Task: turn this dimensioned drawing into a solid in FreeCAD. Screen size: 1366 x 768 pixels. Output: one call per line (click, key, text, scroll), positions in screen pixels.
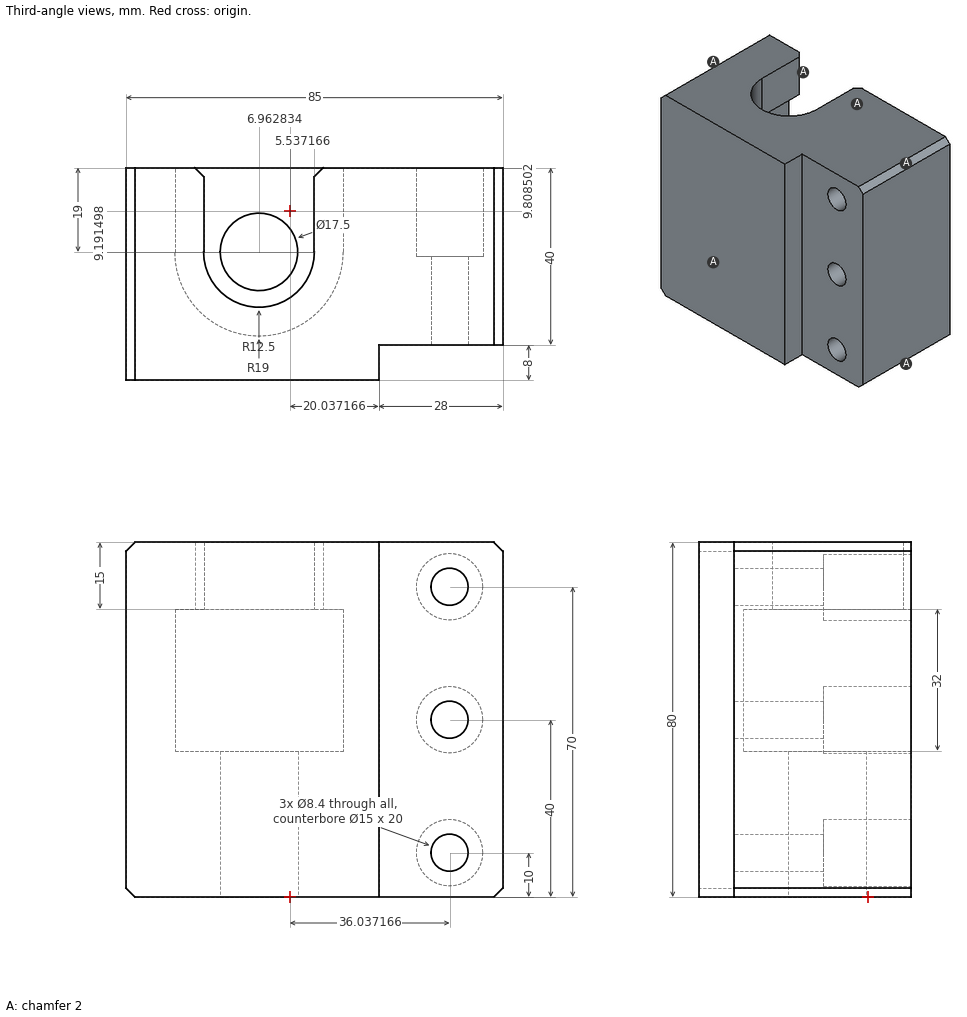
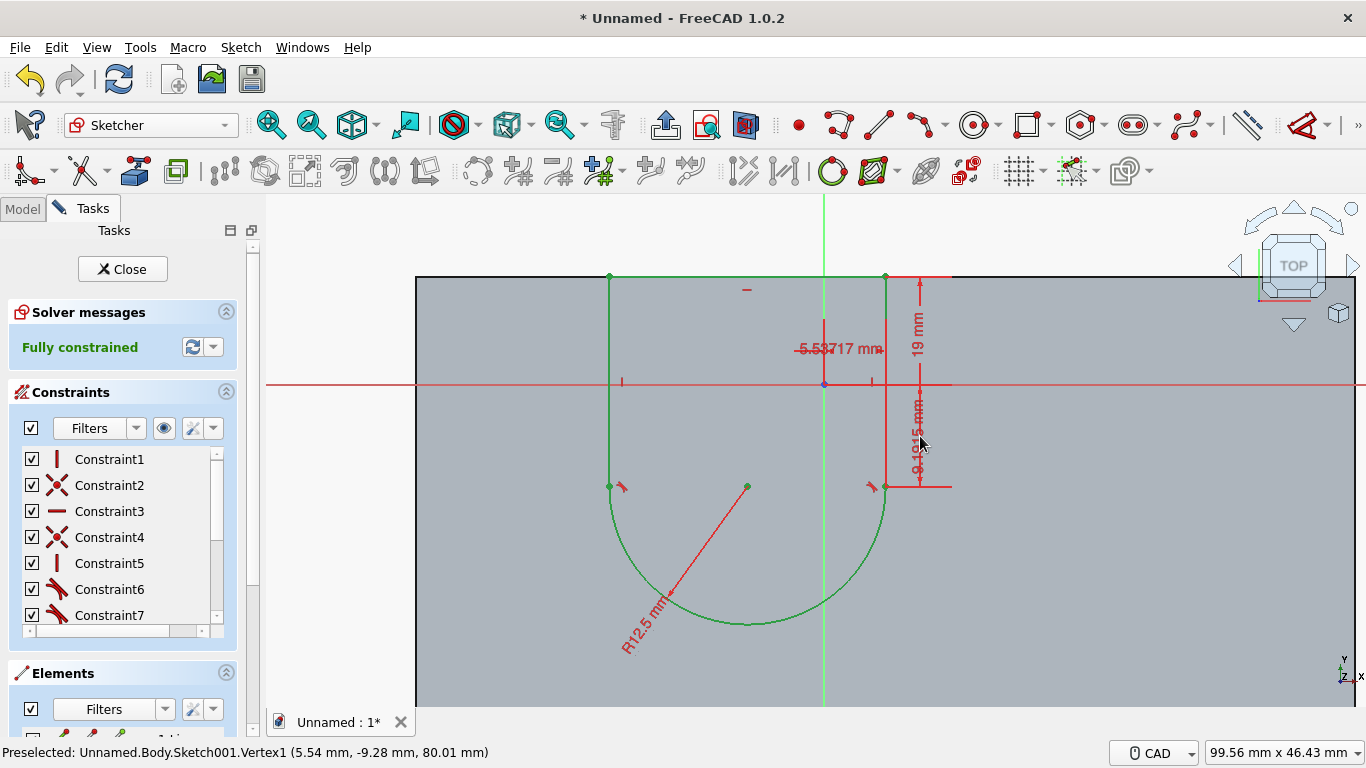
click(123, 269)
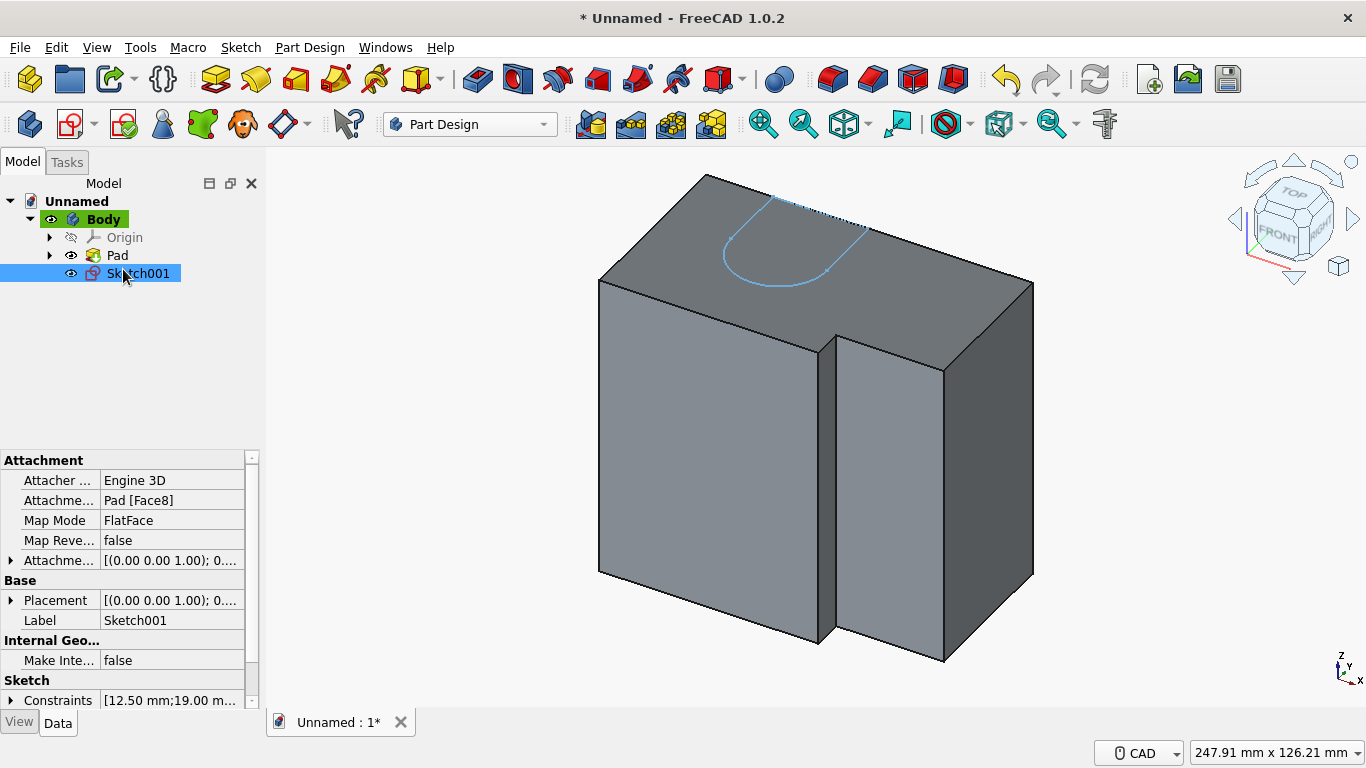
click(478, 80)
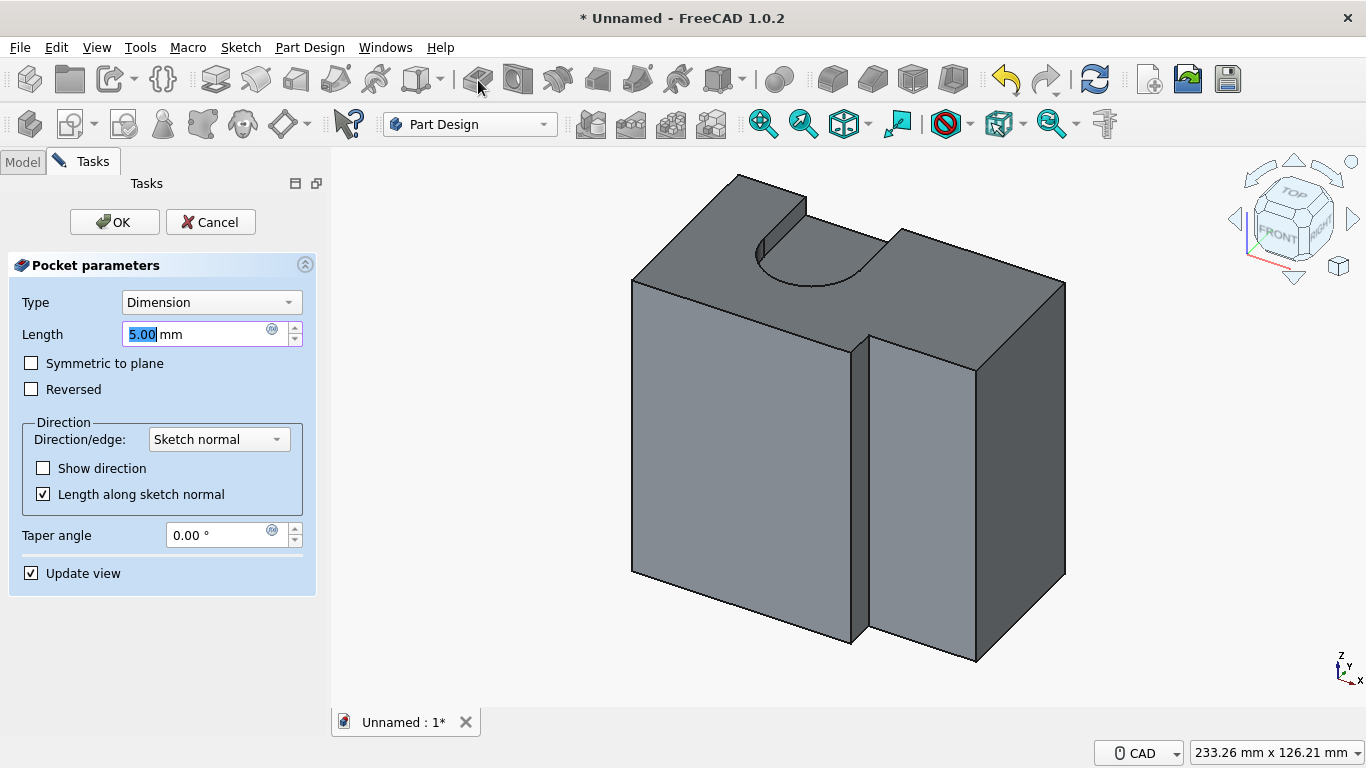
text(15)
key(Tab)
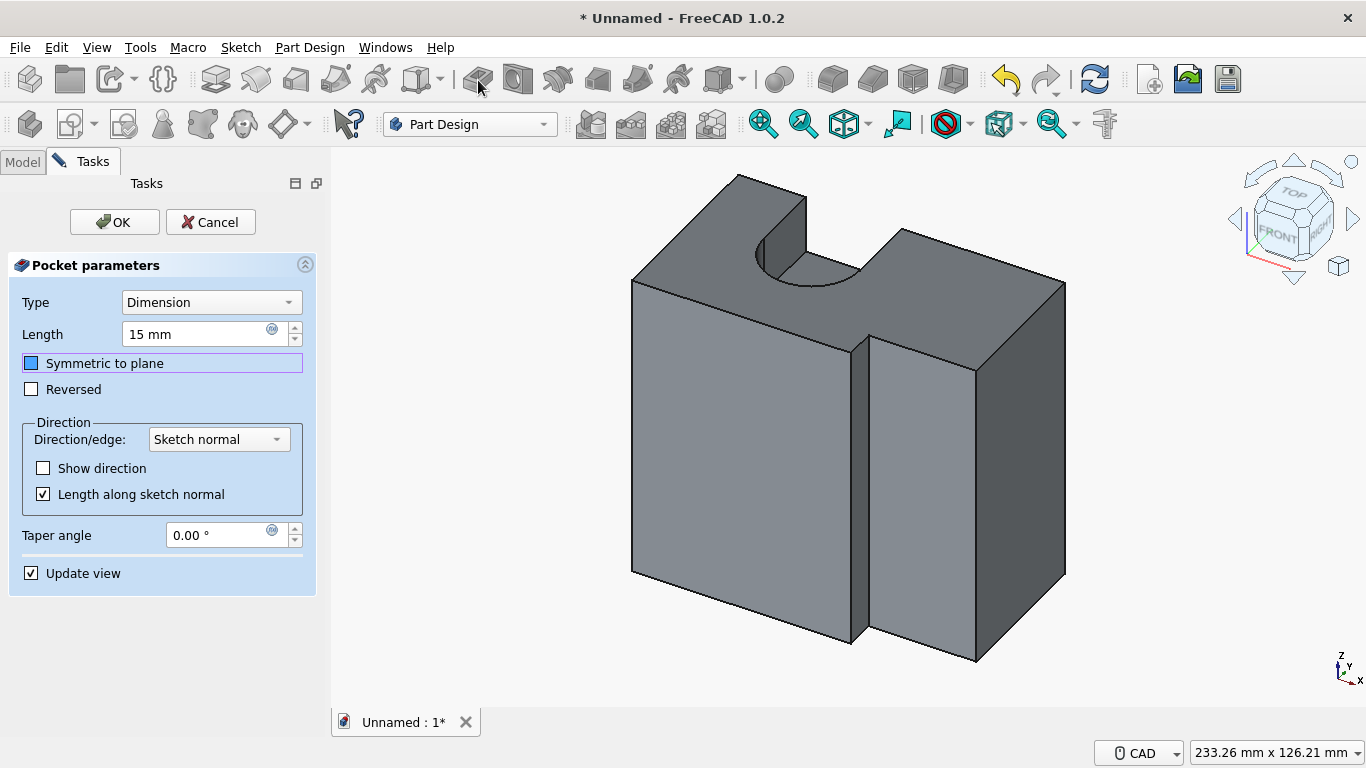
click(115, 222)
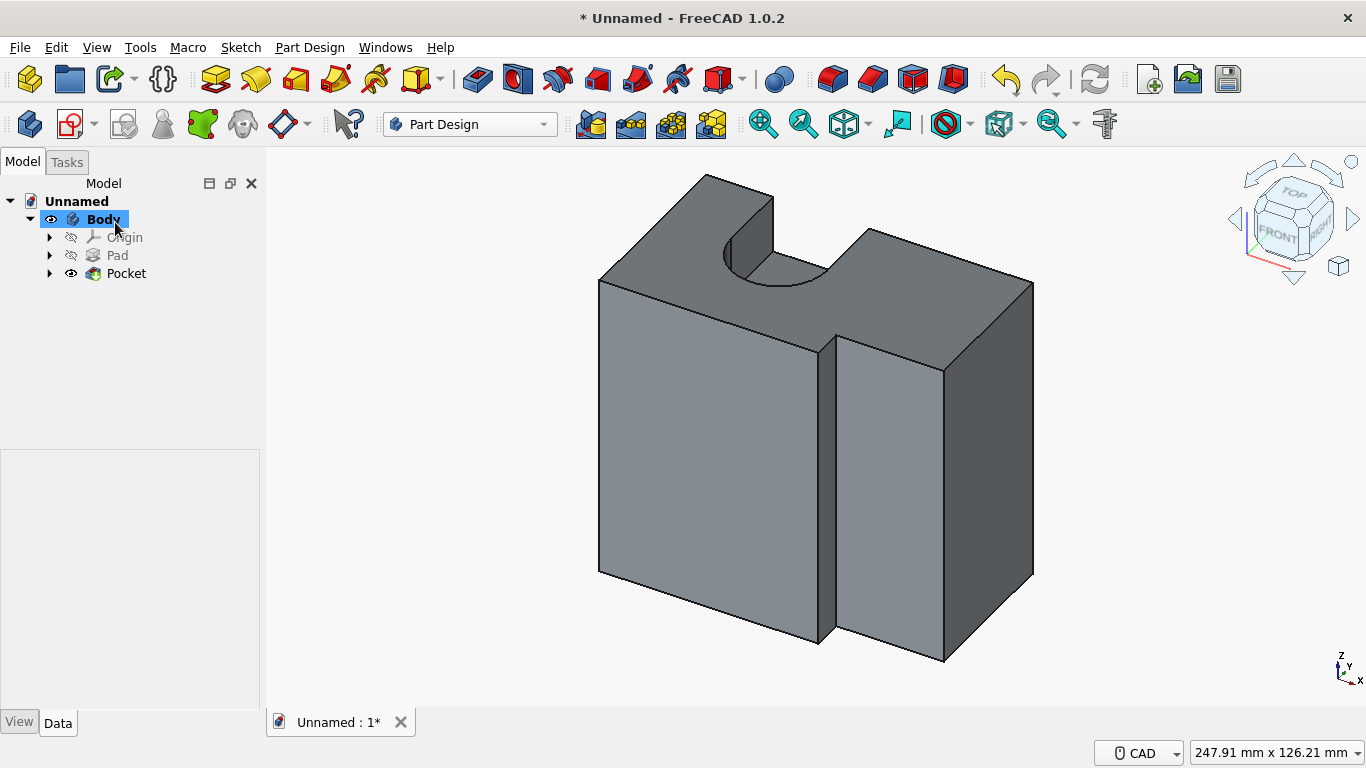
key(0)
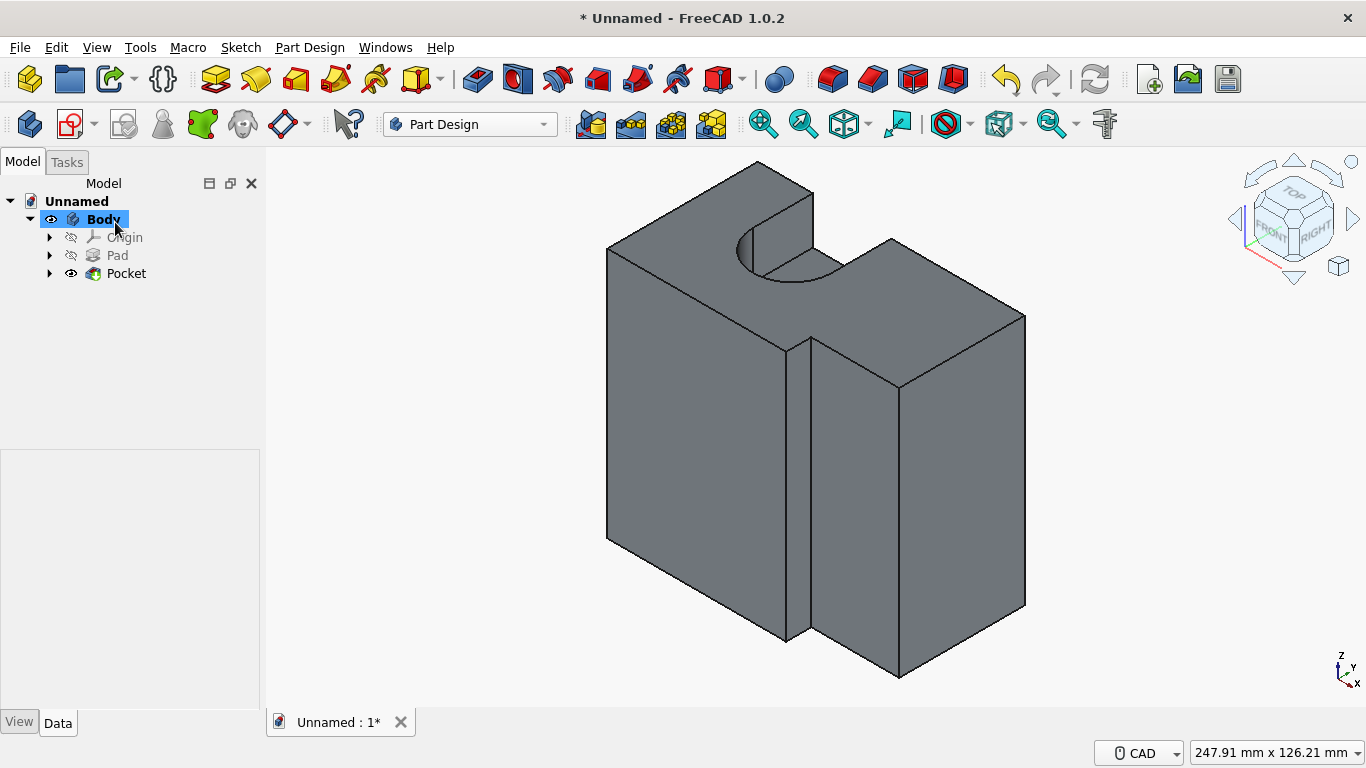
key(2)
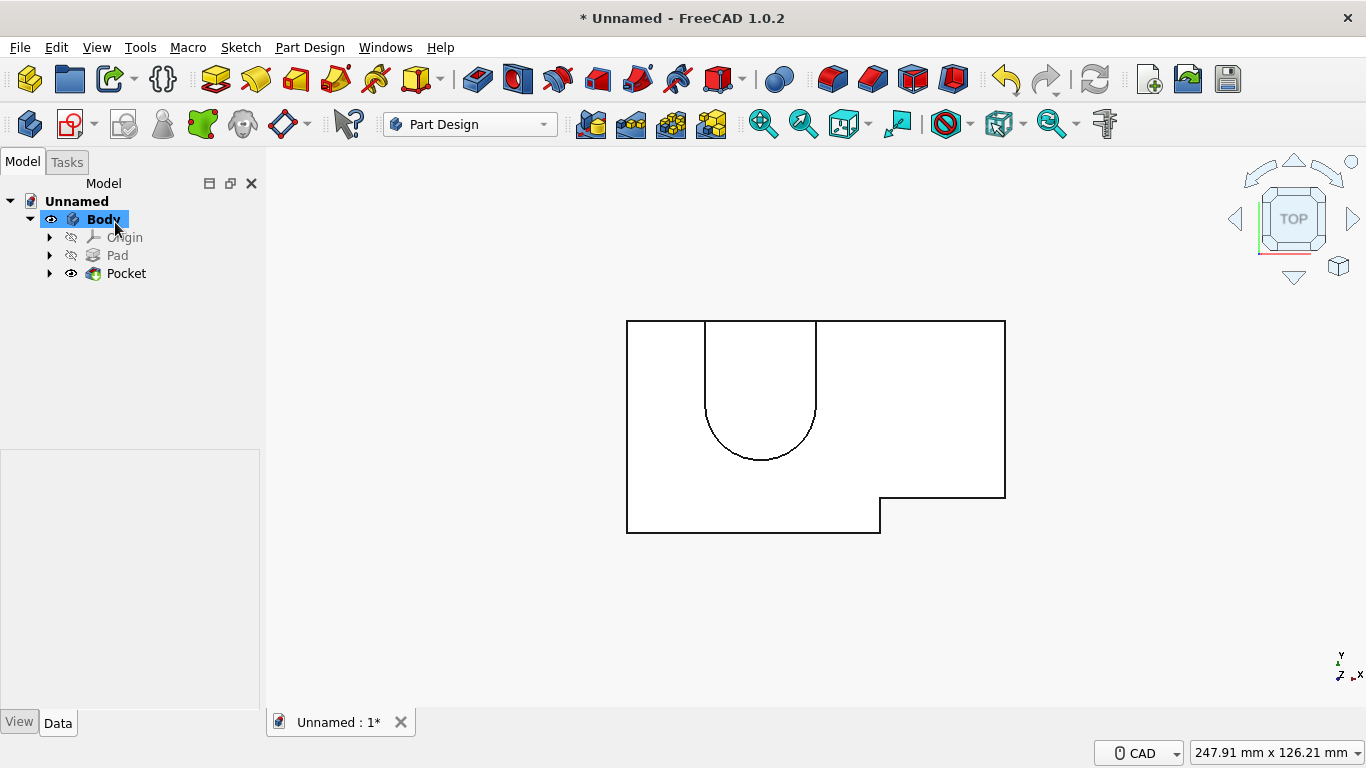
click(764, 124)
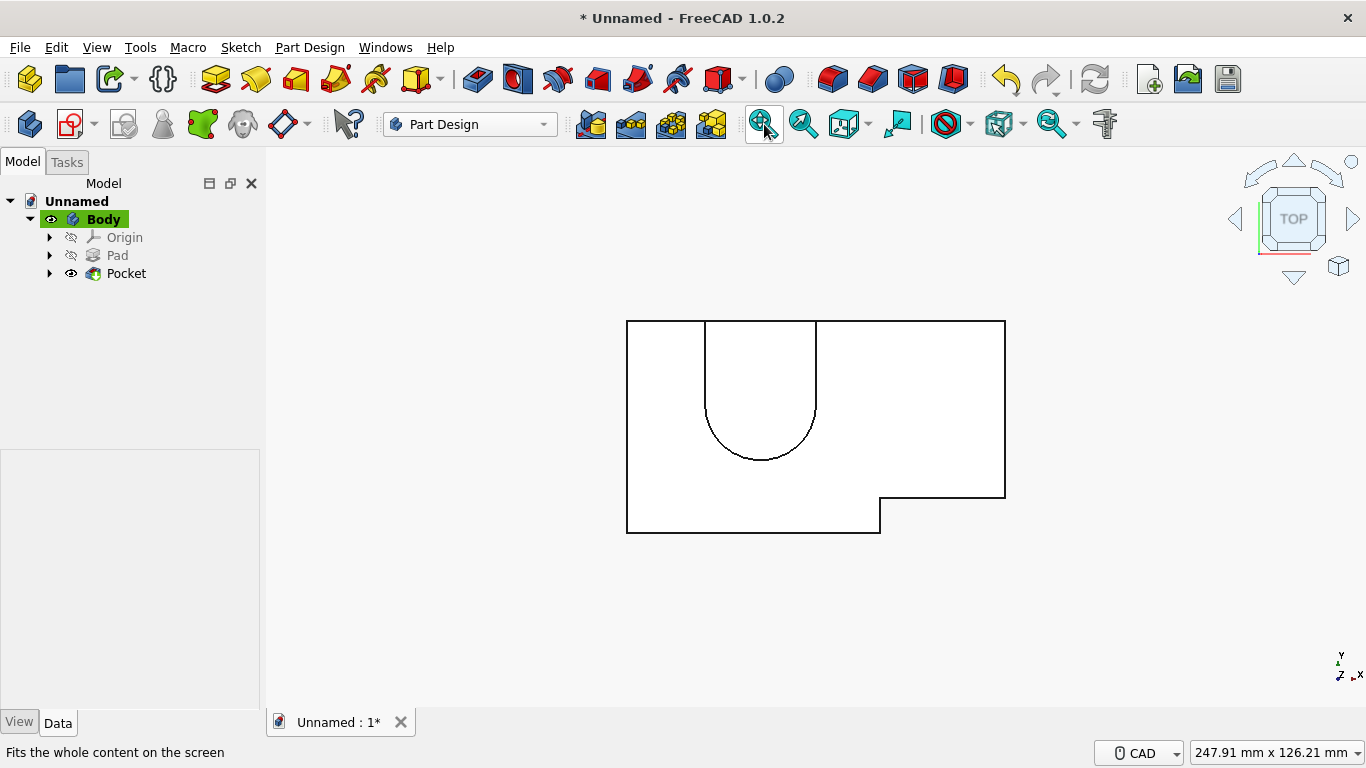
click(761, 389)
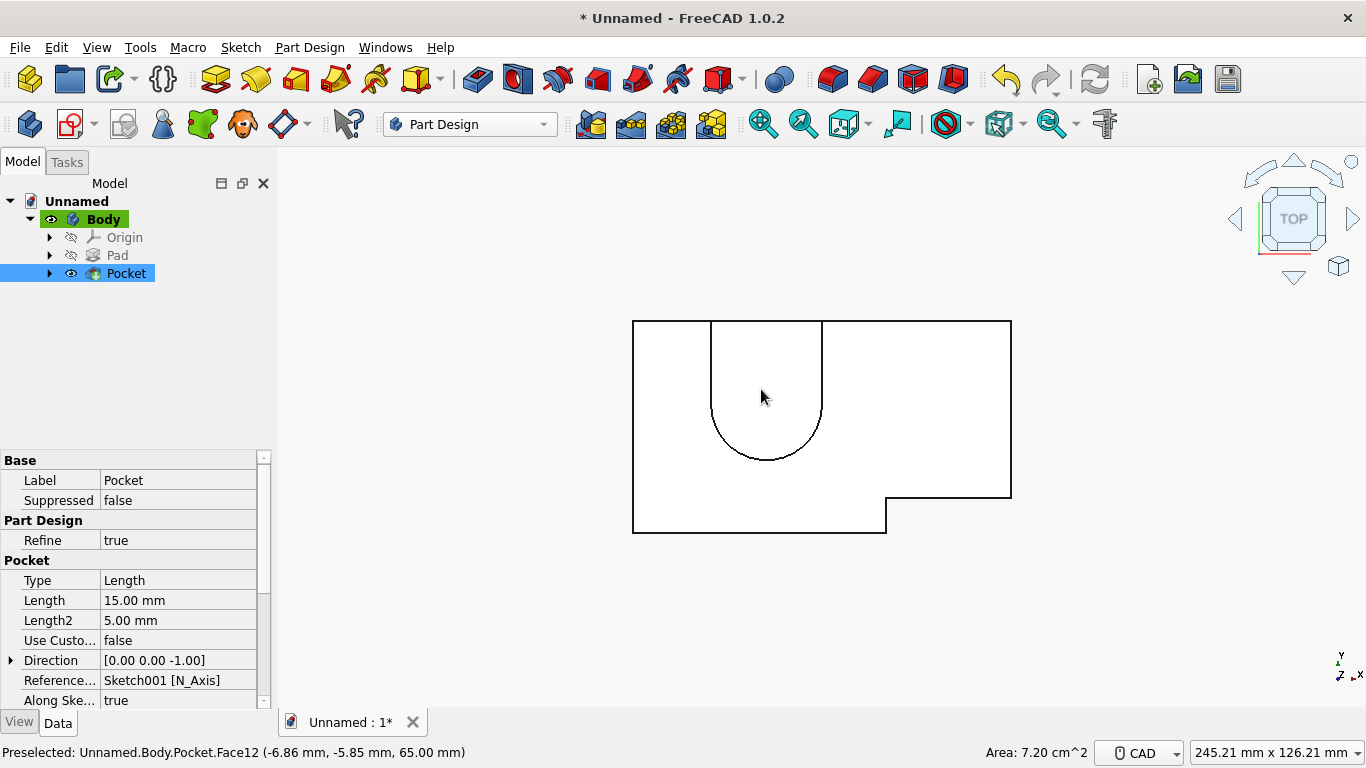
click(70, 124)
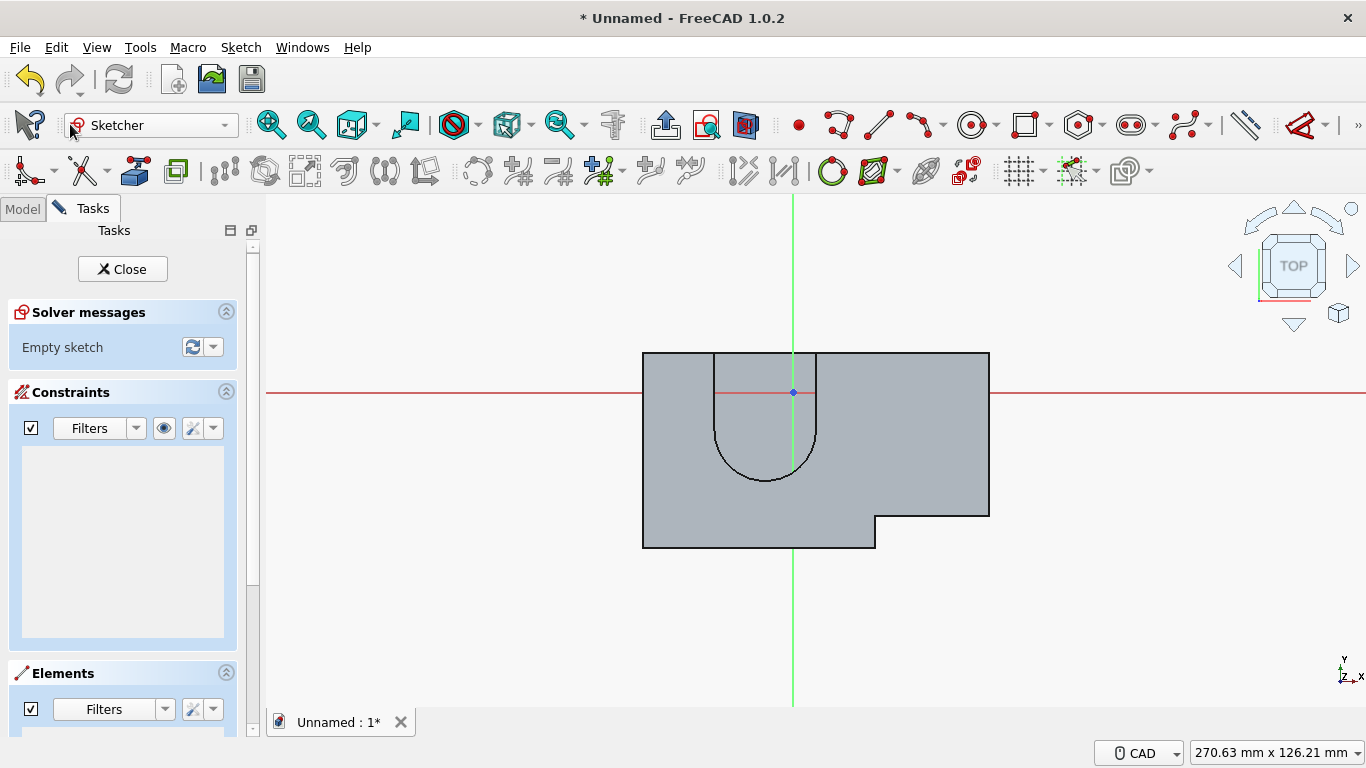
click(746, 126)